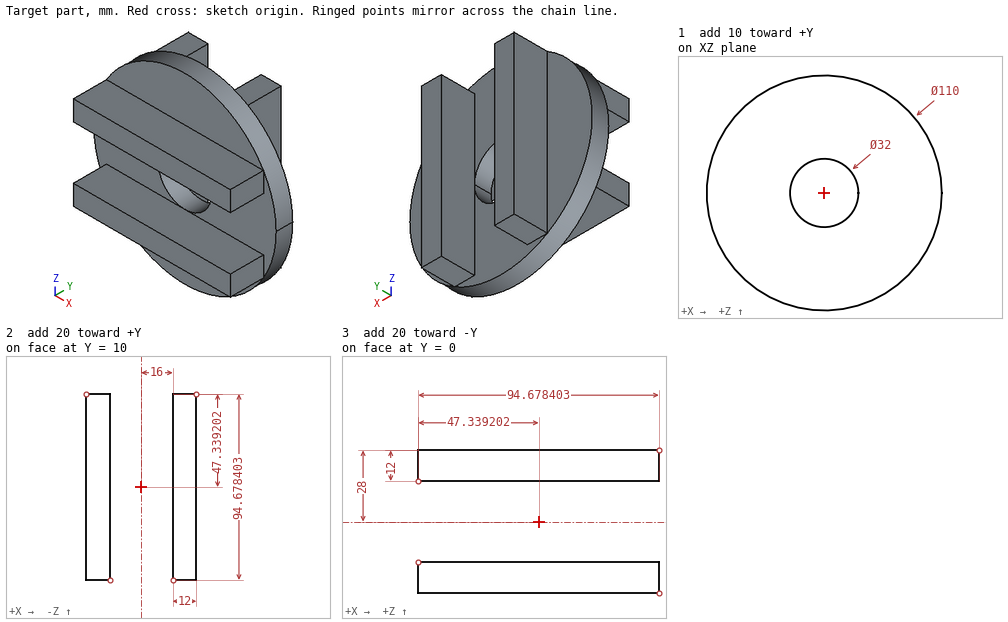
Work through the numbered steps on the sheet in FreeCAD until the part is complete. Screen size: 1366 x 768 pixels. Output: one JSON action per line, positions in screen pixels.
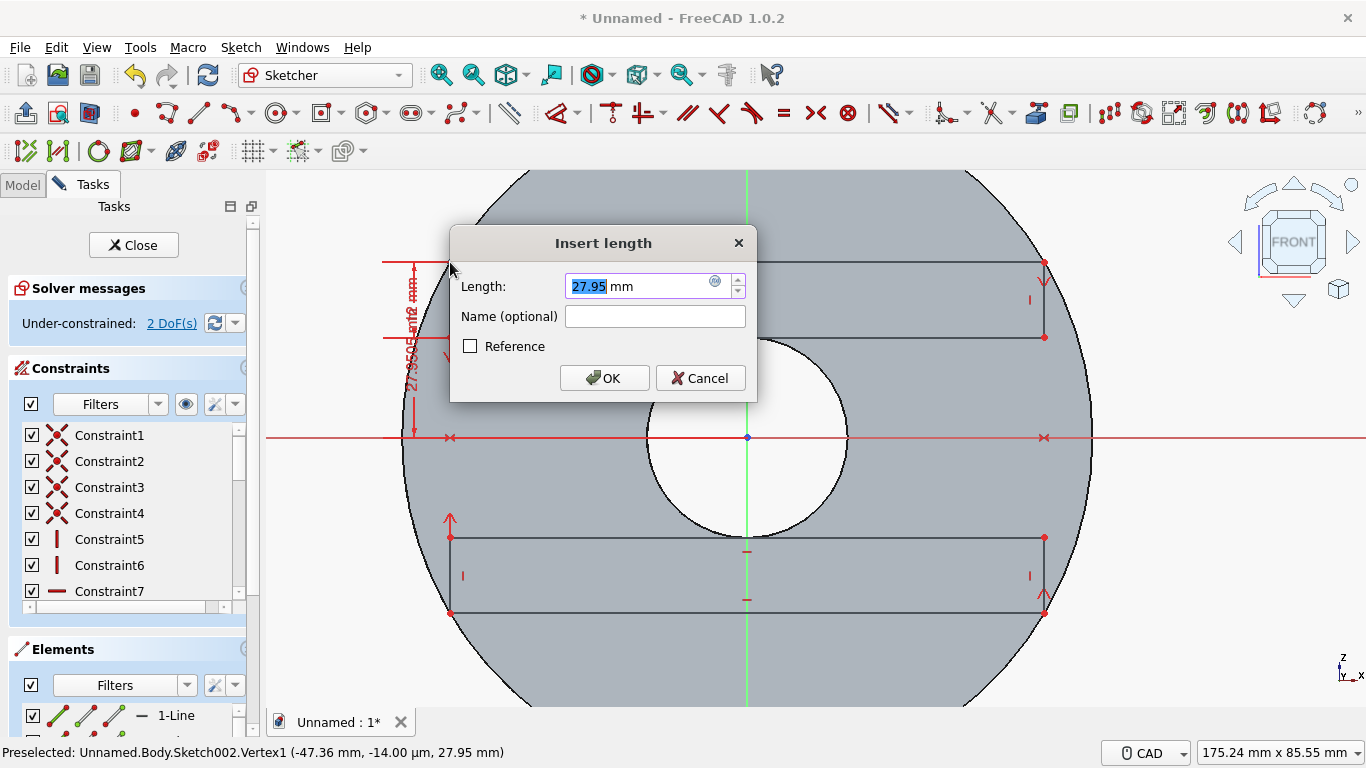
{"action": "type", "text": "28"}
{"action": "key", "text": "Return"}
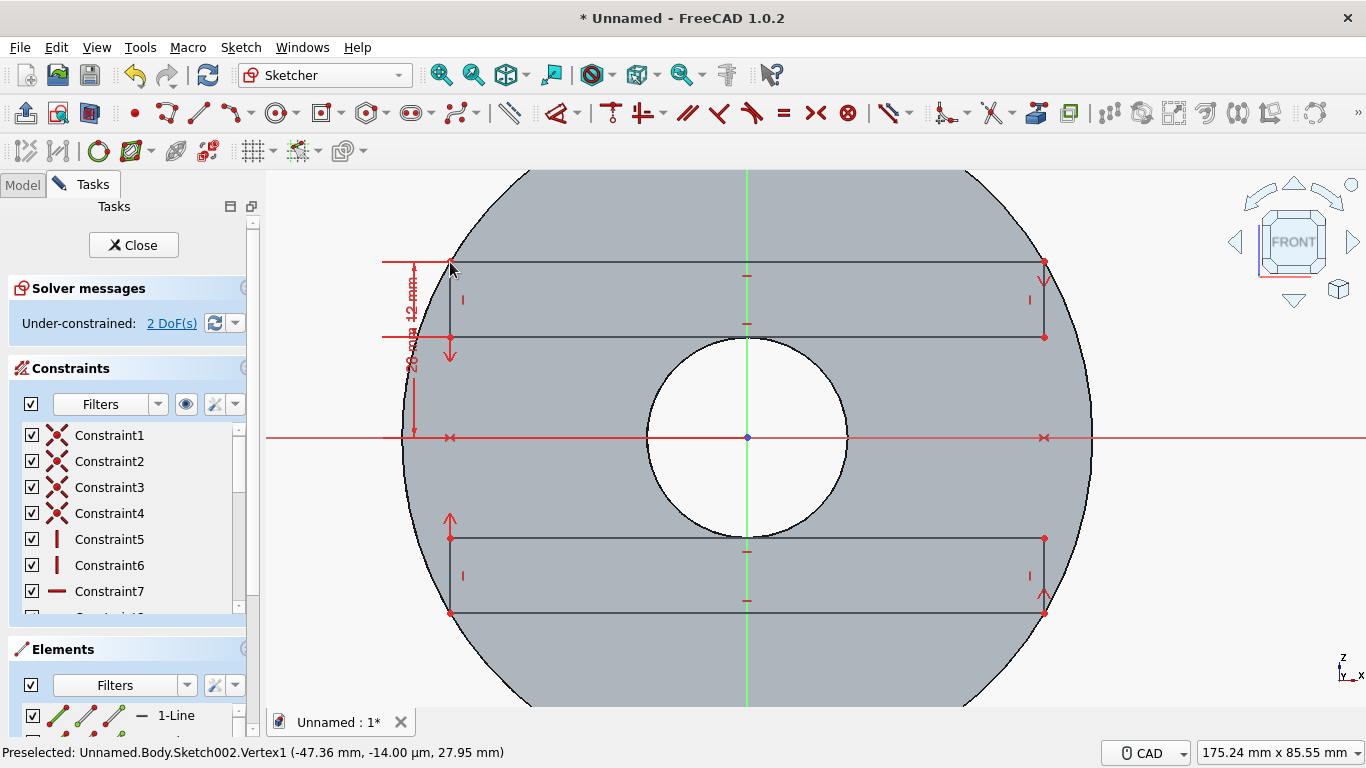
{"action": "left_click", "coordinate": [628, 337]}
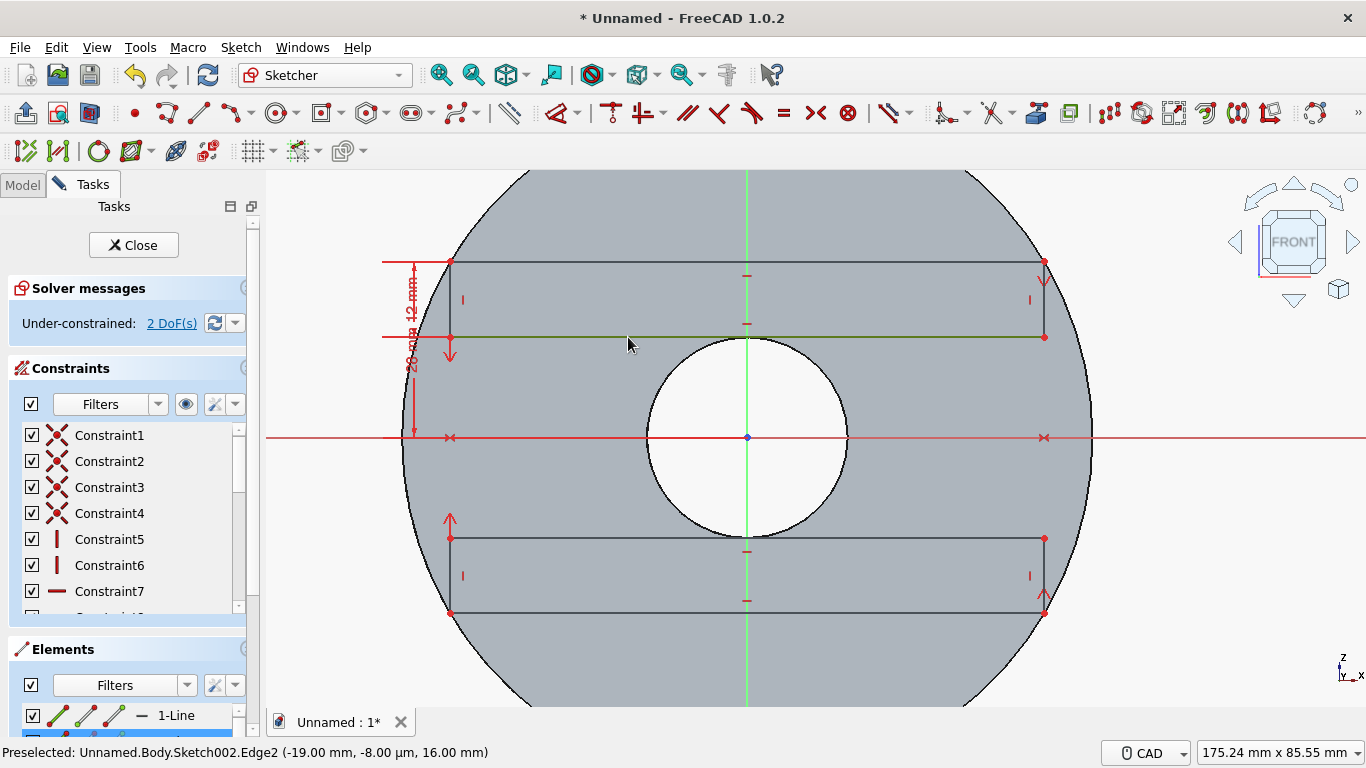
{"action": "key", "text": "l"}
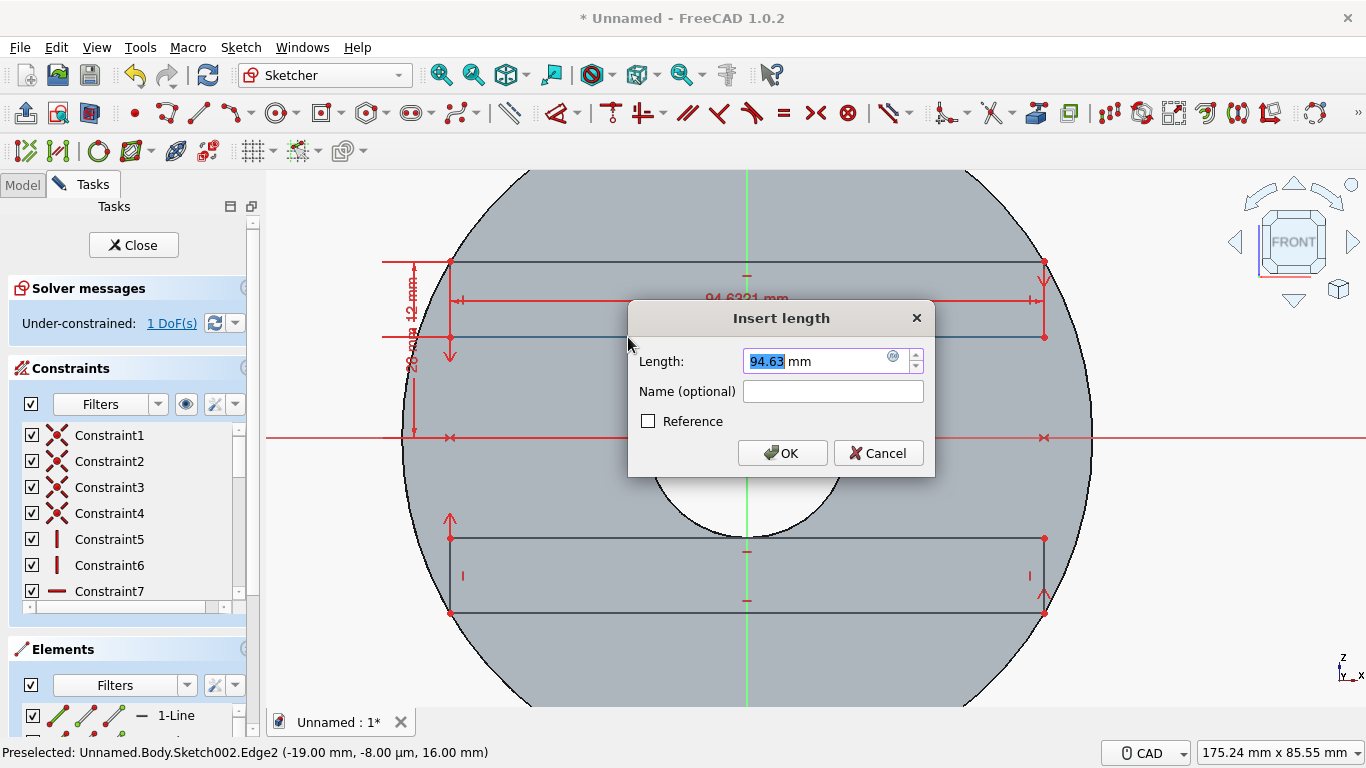
{"action": "type", "text": "94.678403"}
{"action": "key", "text": "Return"}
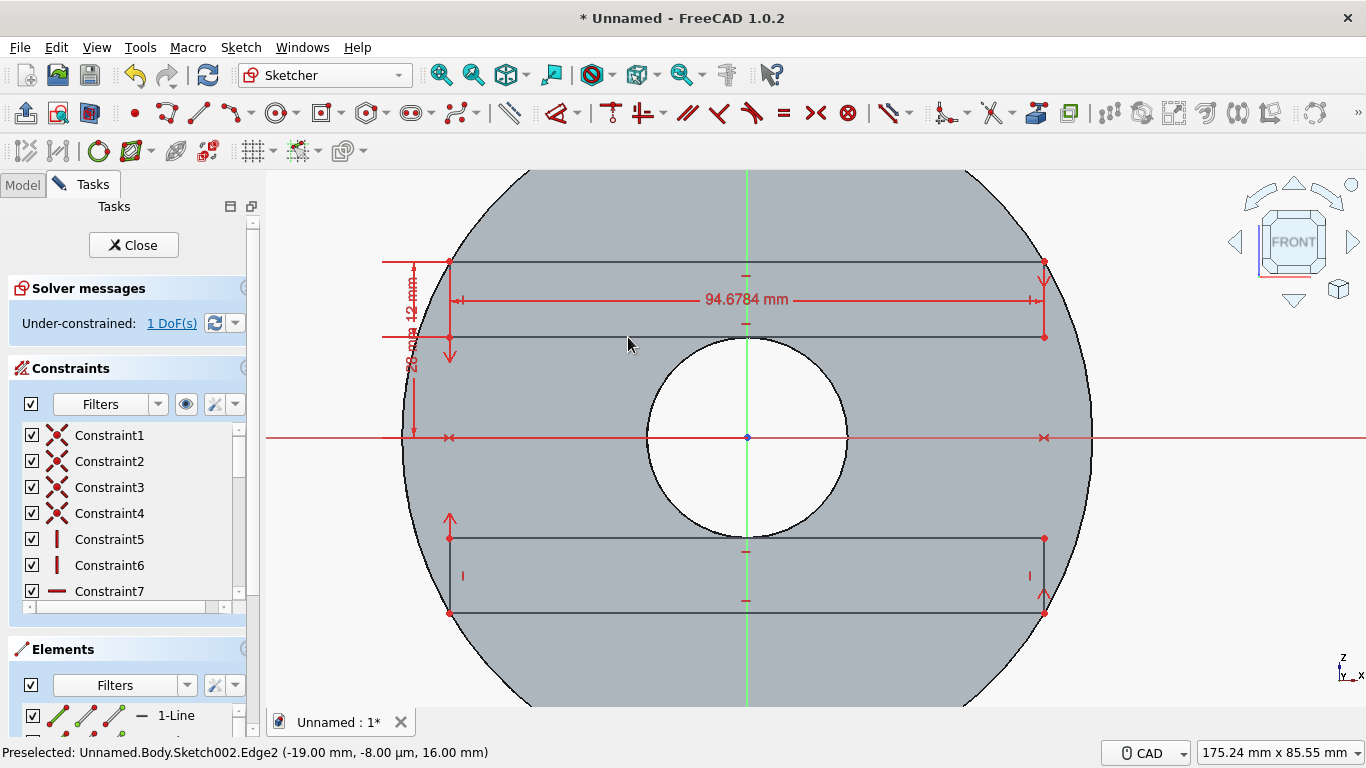
{"action": "left_click", "coordinate": [450, 262]}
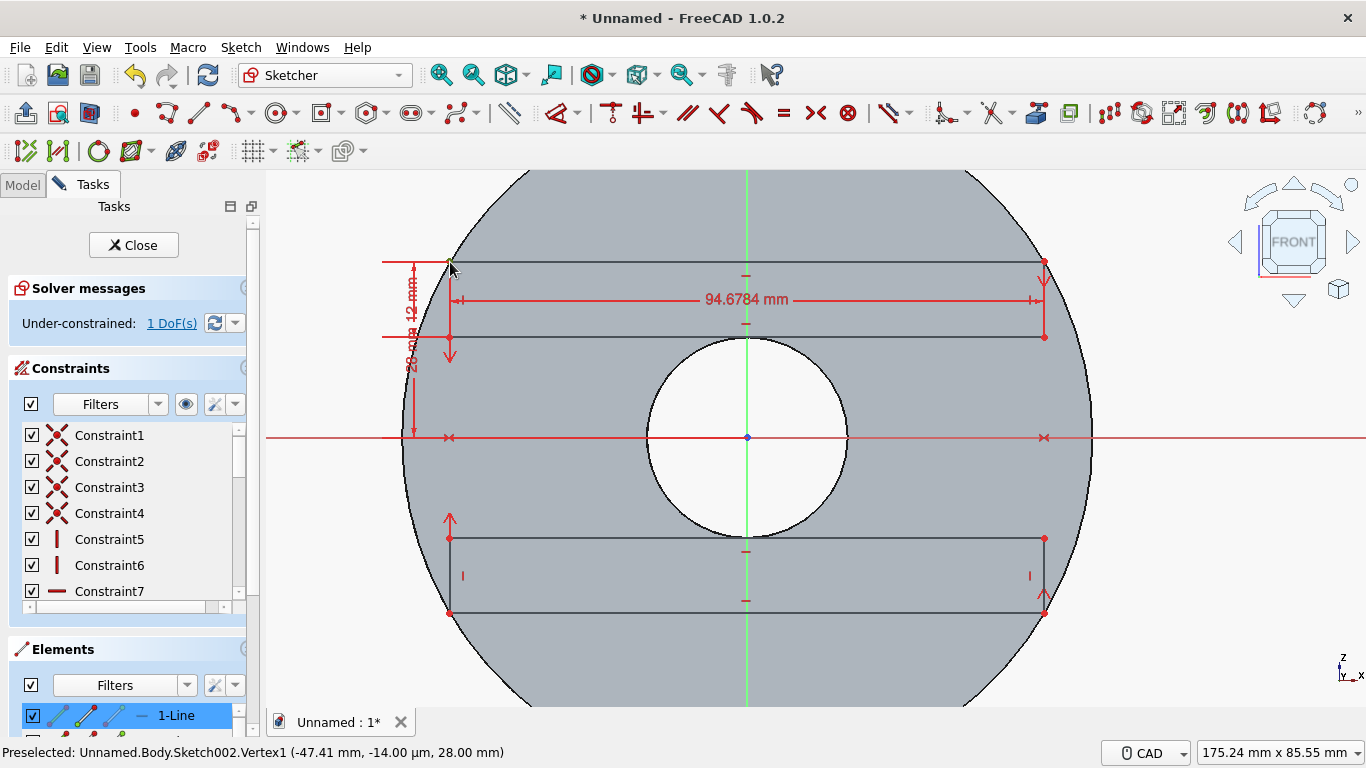
{"action": "key", "text": "l"}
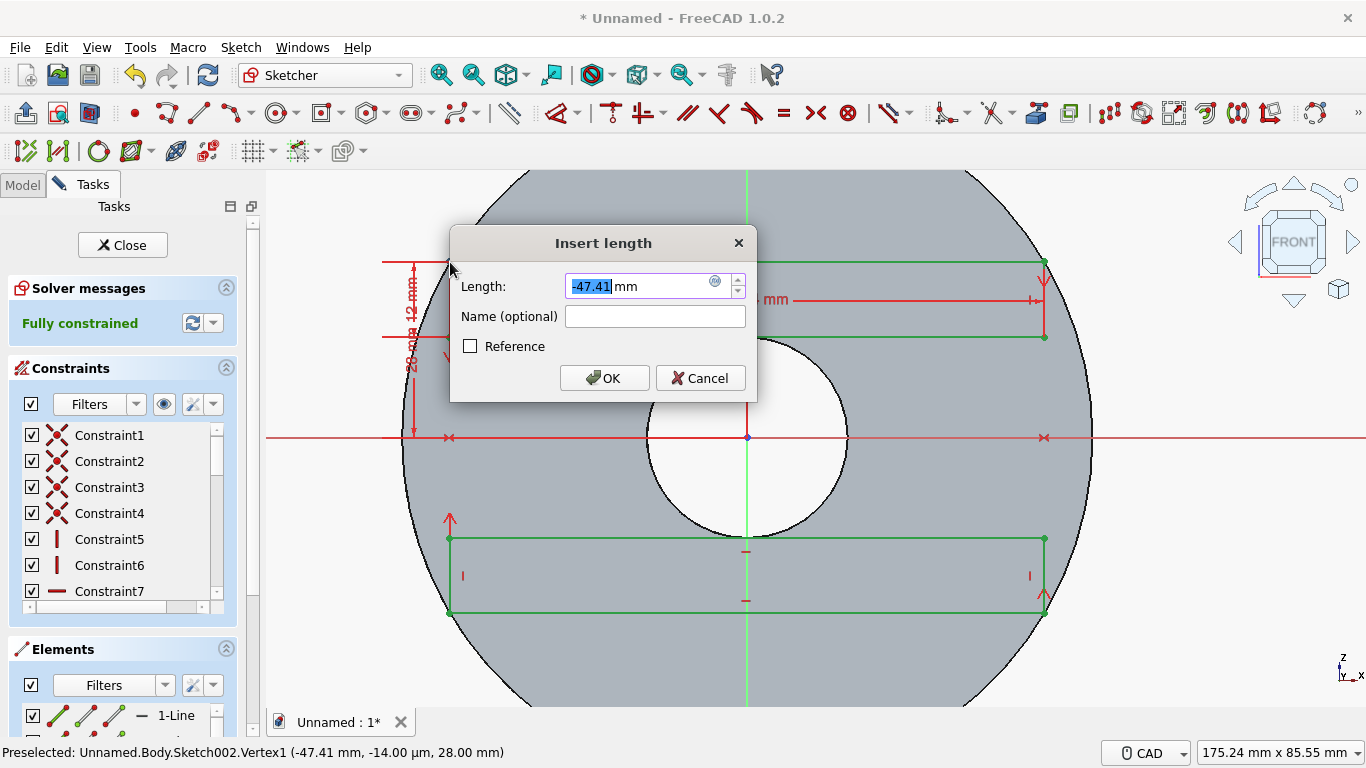
{"action": "type", "text": "-47.339202"}
{"action": "key", "text": "Return"}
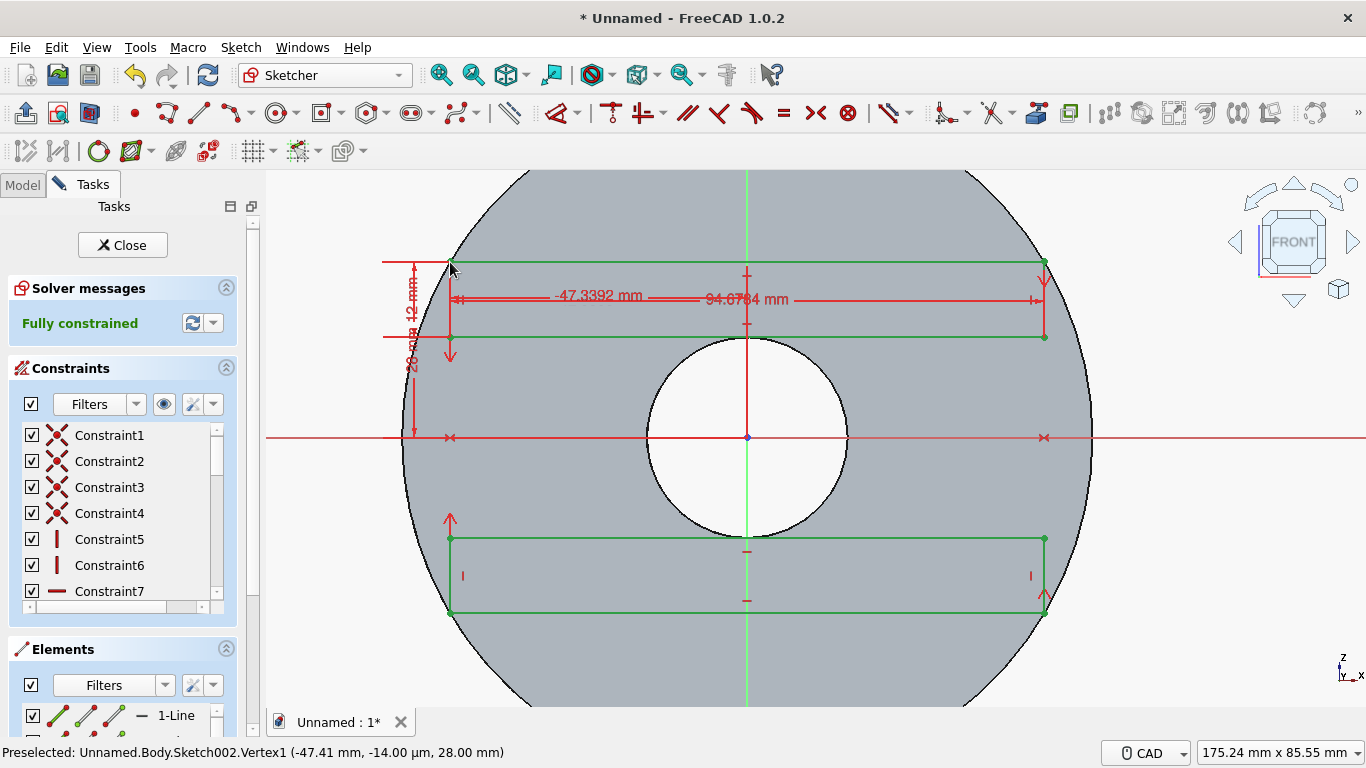
{"action": "left_click", "coordinate": [123, 245]}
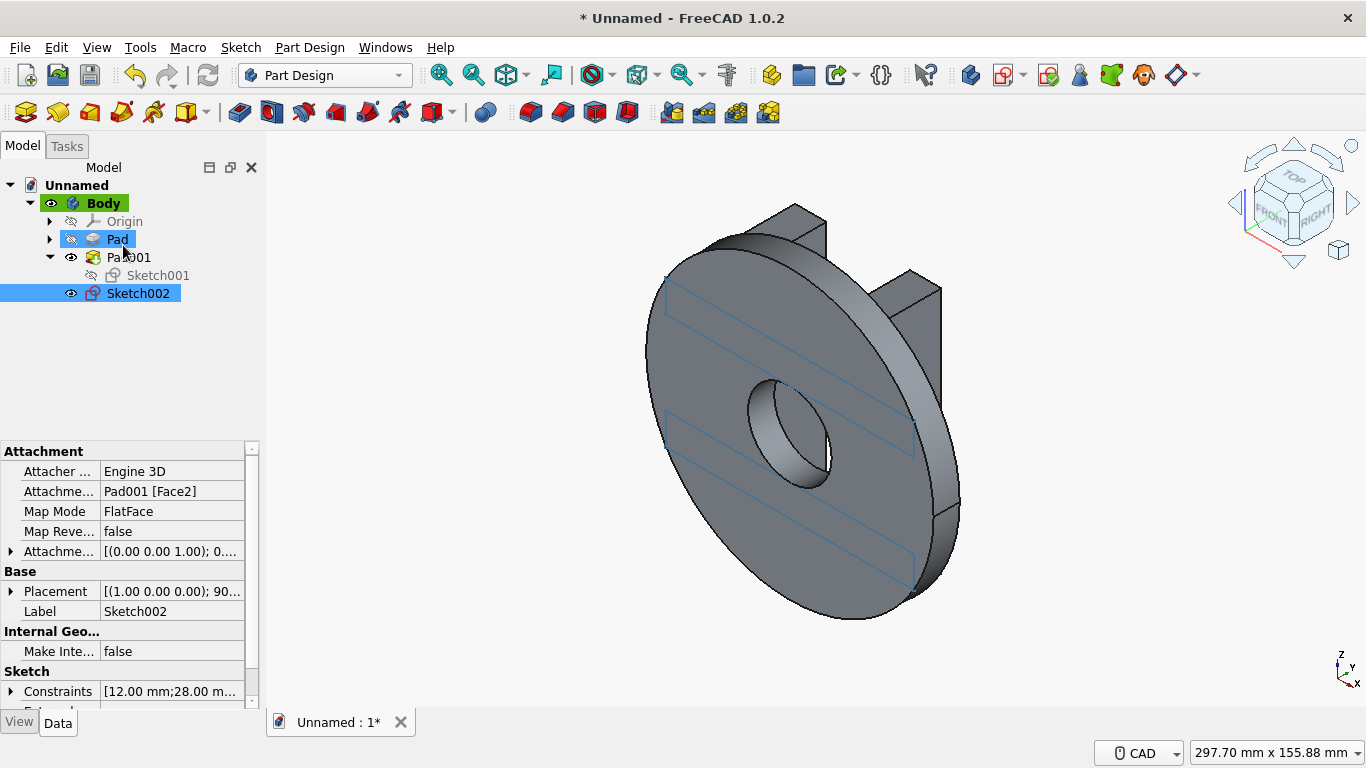
{"action": "left_click", "coordinate": [26, 112]}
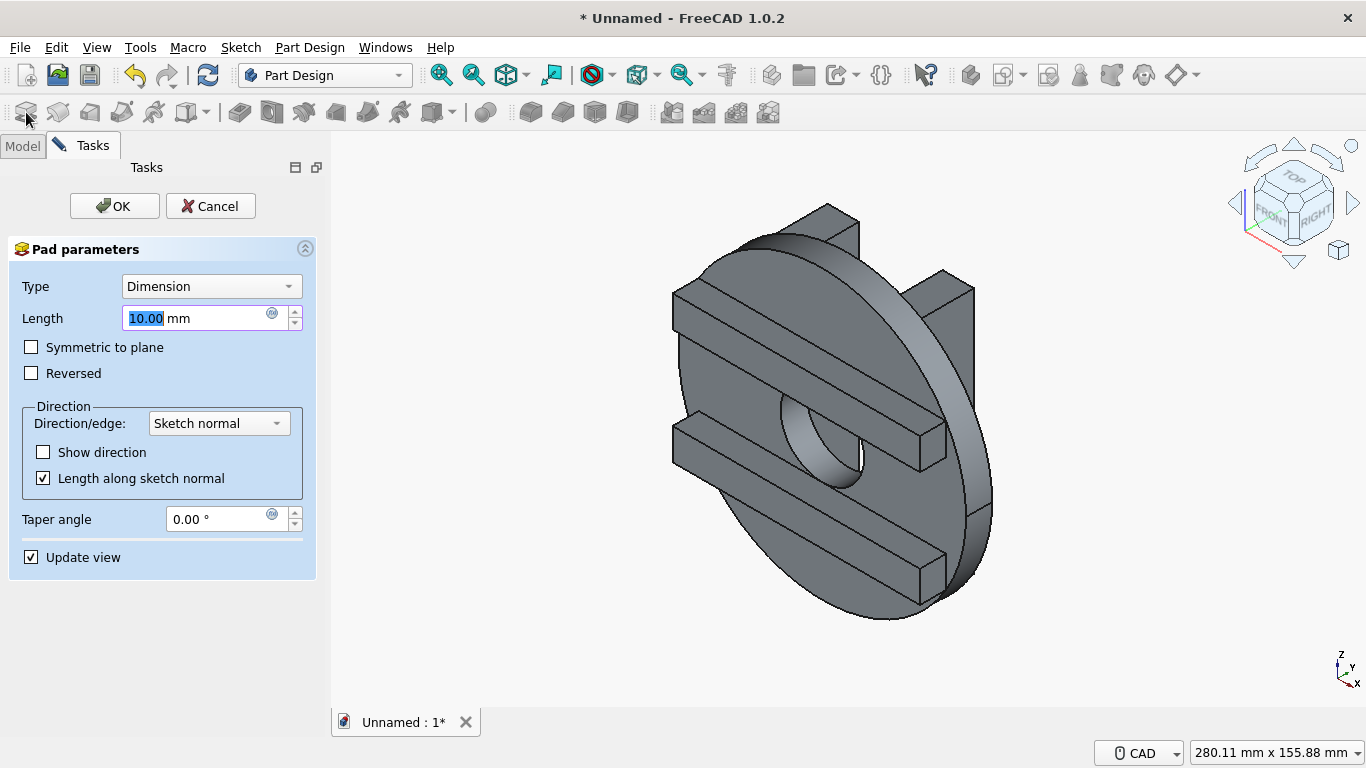
{"action": "type", "text": "20"}
{"action": "key", "text": "Tab"}